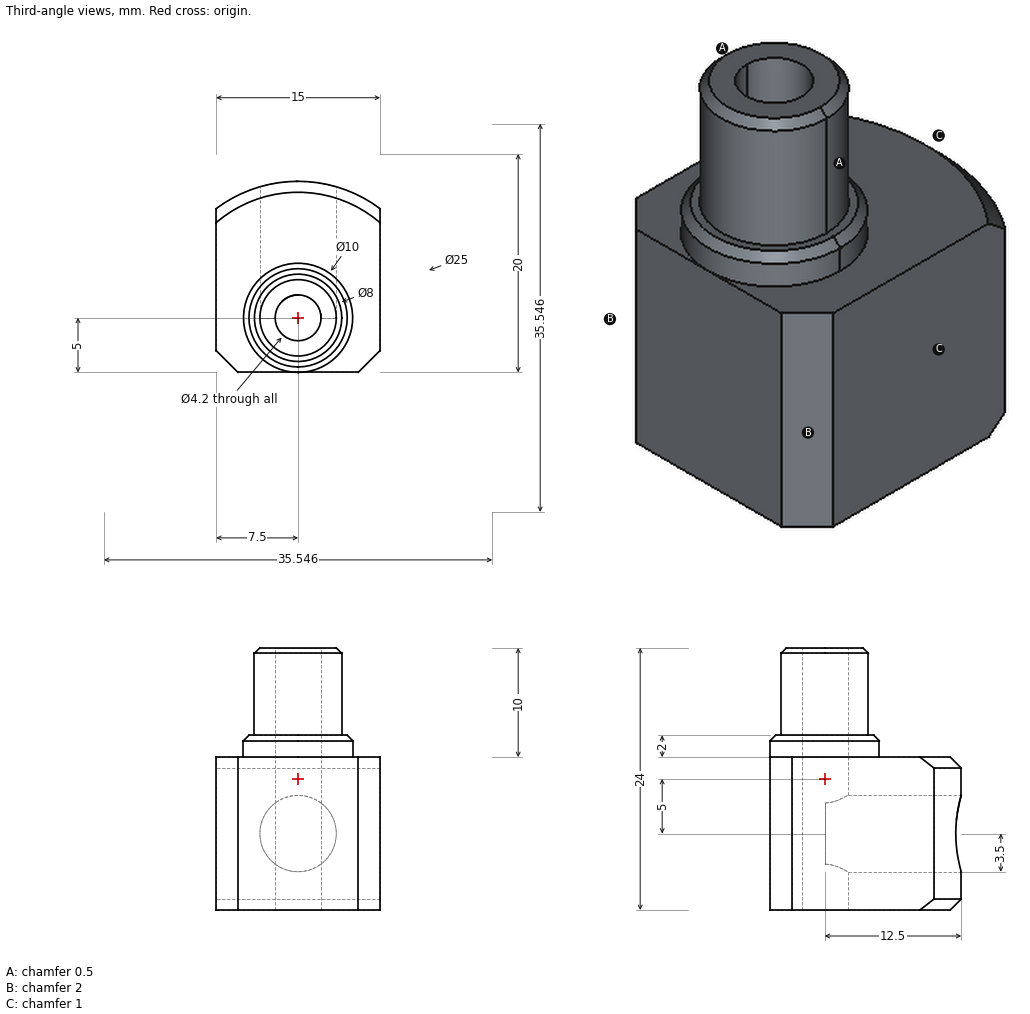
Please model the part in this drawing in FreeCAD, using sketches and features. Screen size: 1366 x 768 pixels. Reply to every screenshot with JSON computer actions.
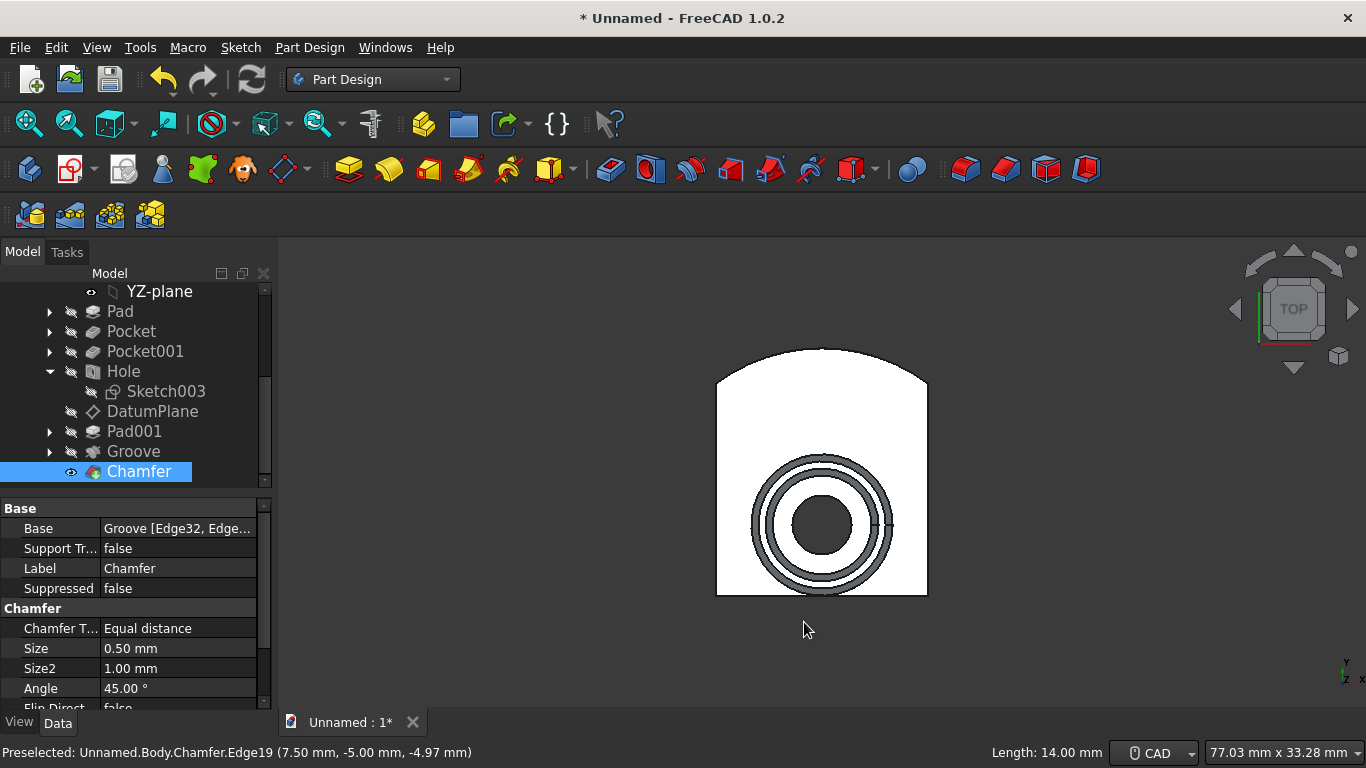
{"action": "key", "text": "0"}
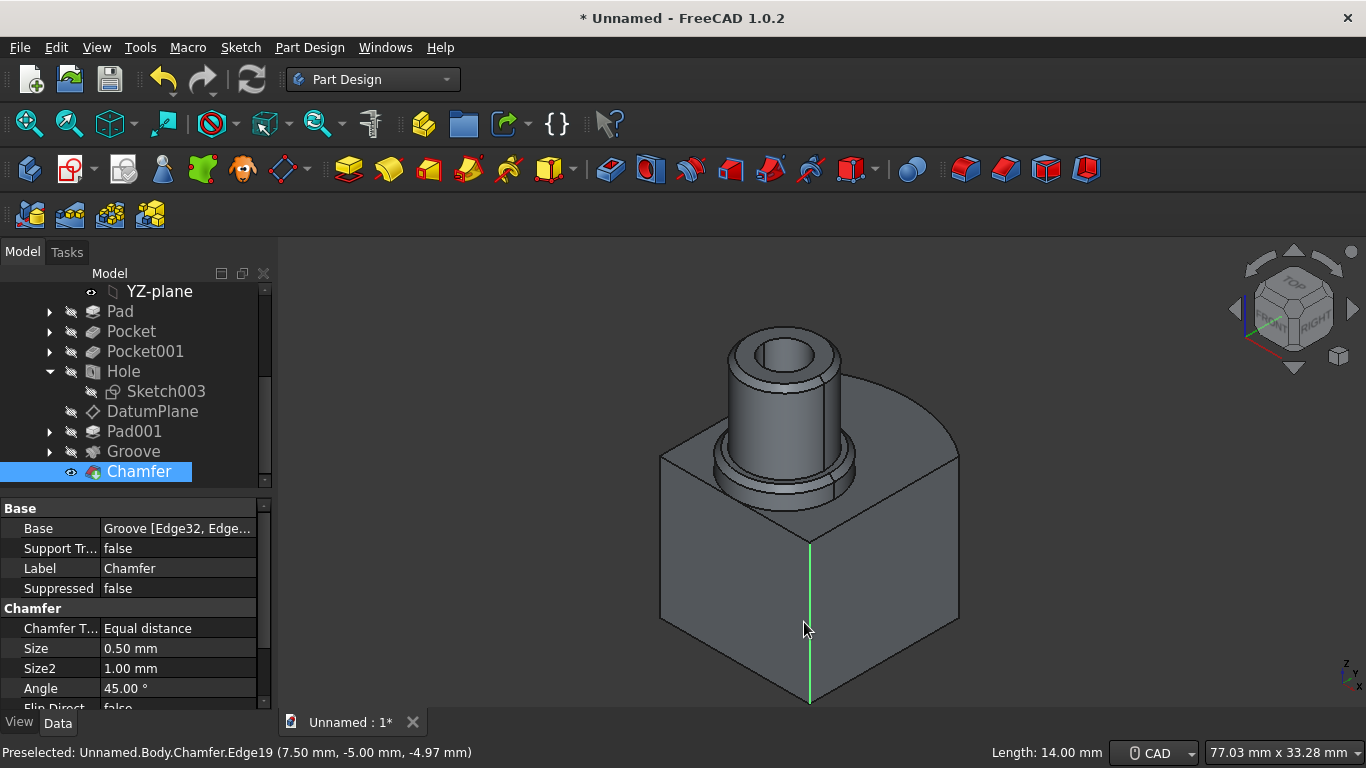
{"action": "key", "text": "1"}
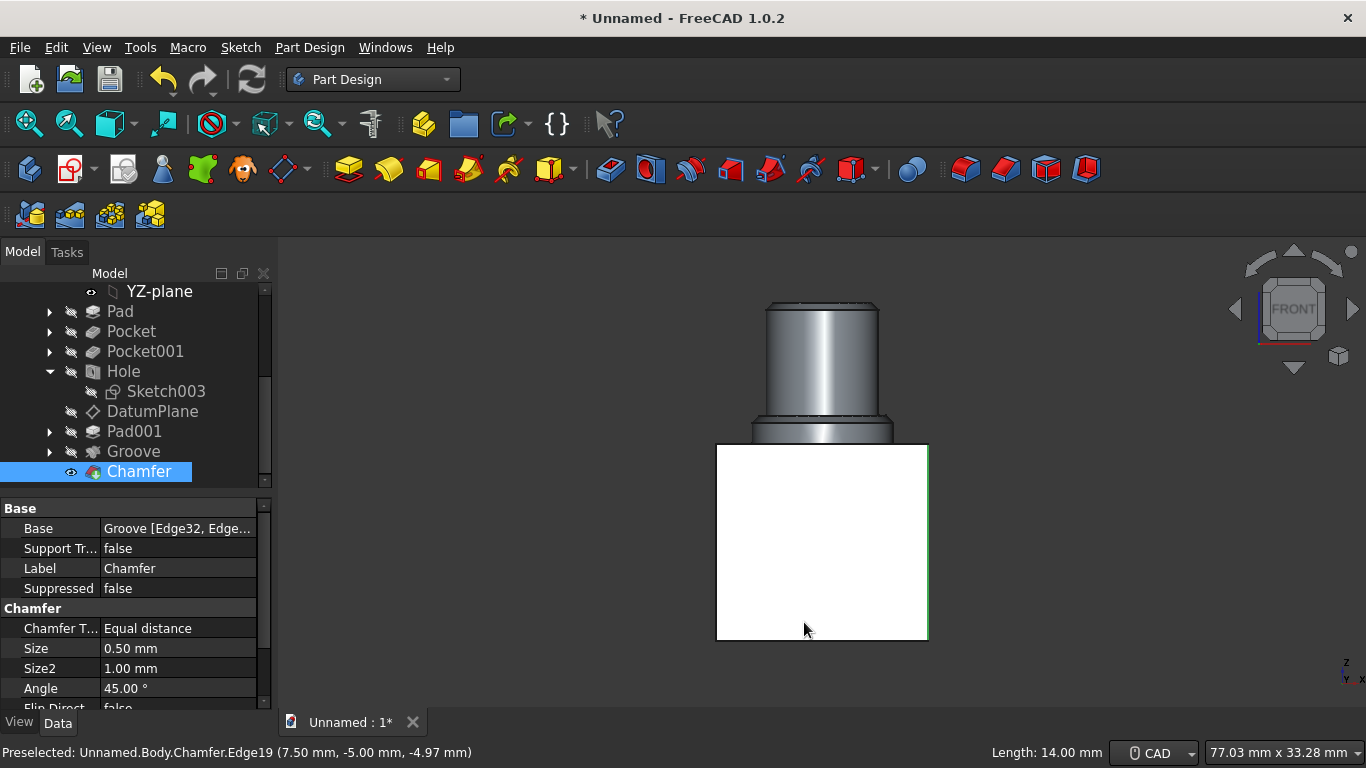
{"action": "left_click", "coordinate": [716, 542], "text": "ctrl"}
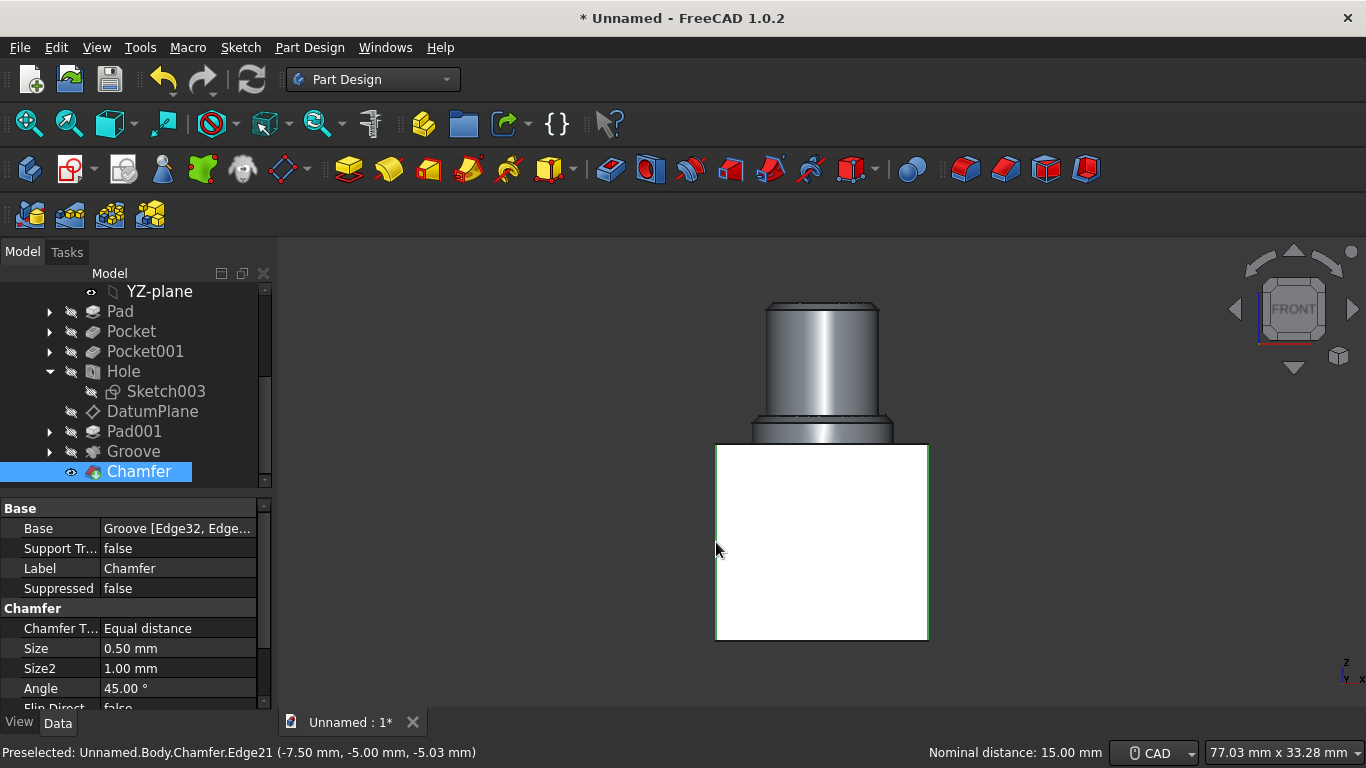
{"action": "left_click", "coordinate": [1006, 170]}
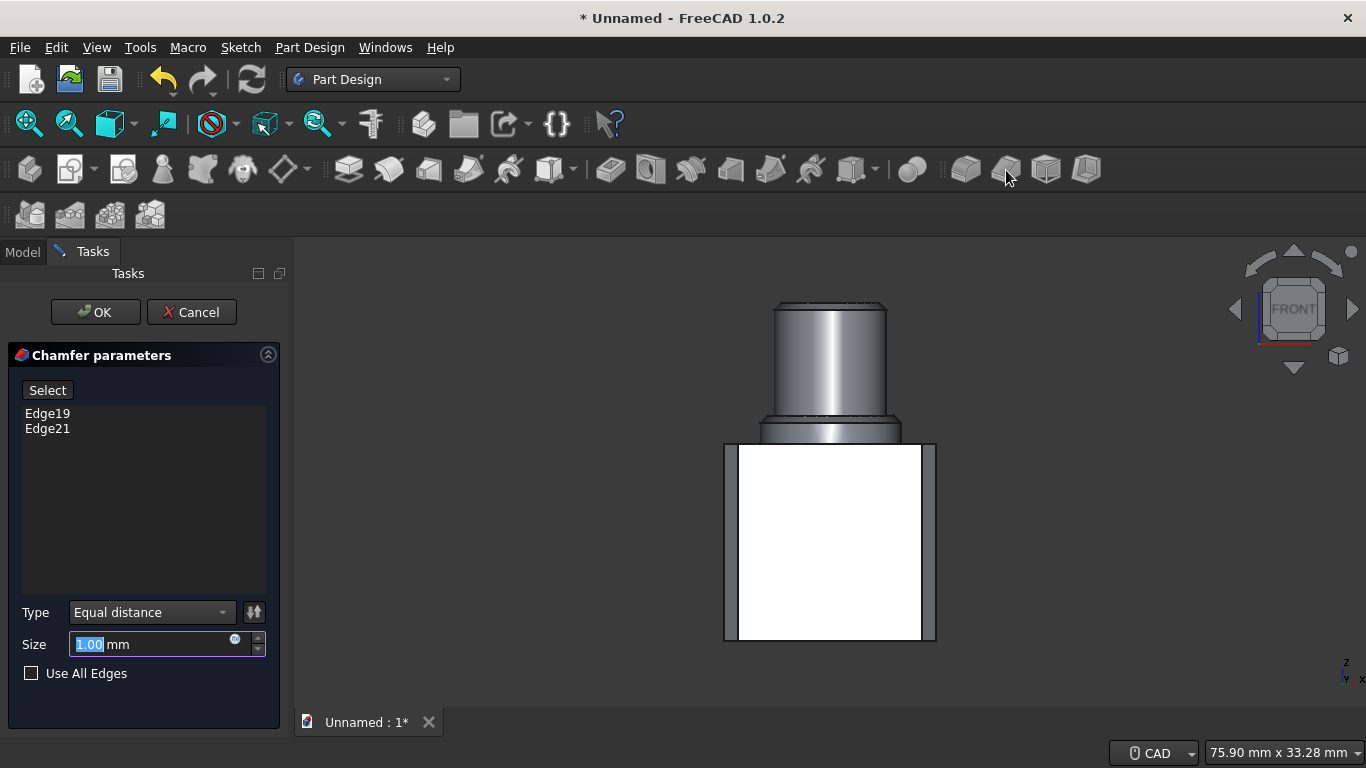
{"action": "type", "text": "2"}
{"action": "key", "text": "Tab"}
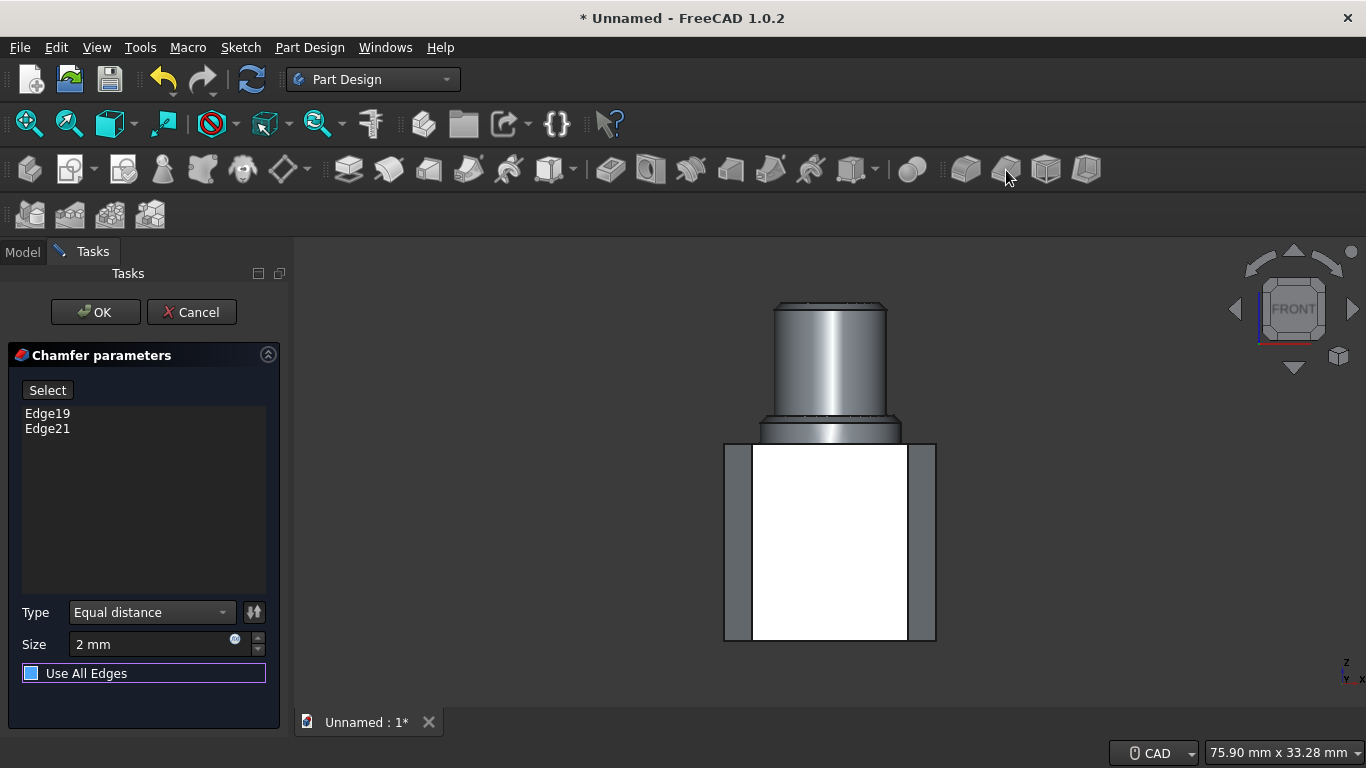
{"action": "left_click", "coordinate": [96, 312]}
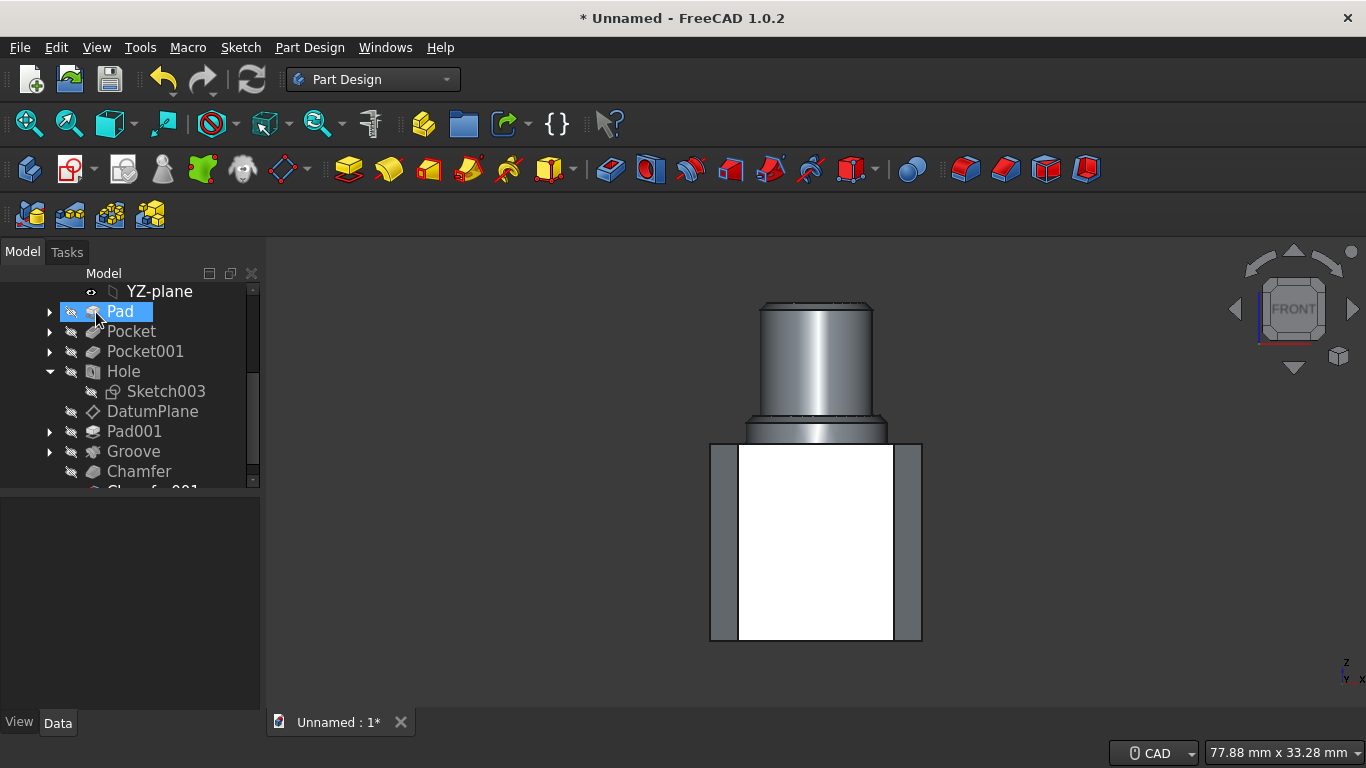
{"action": "key", "text": "0"}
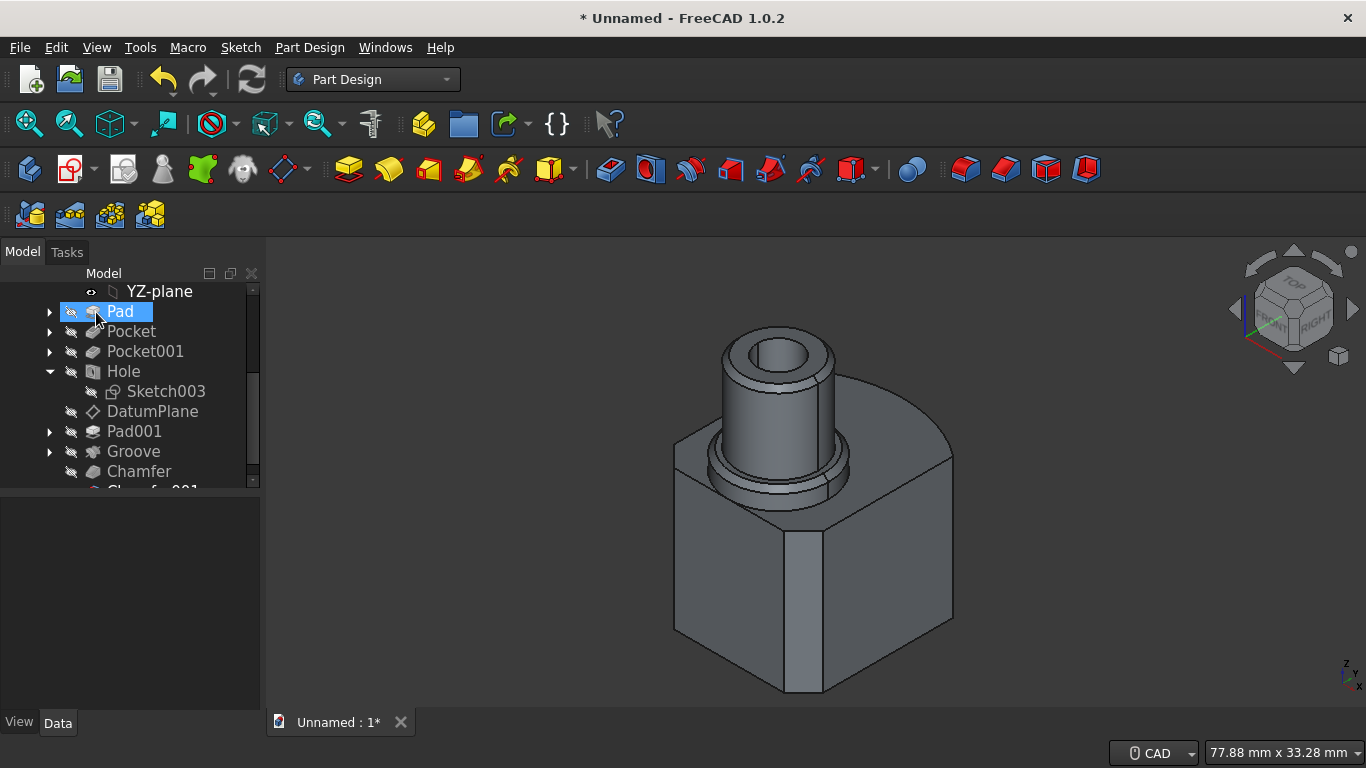
{"action": "key", "text": "2"}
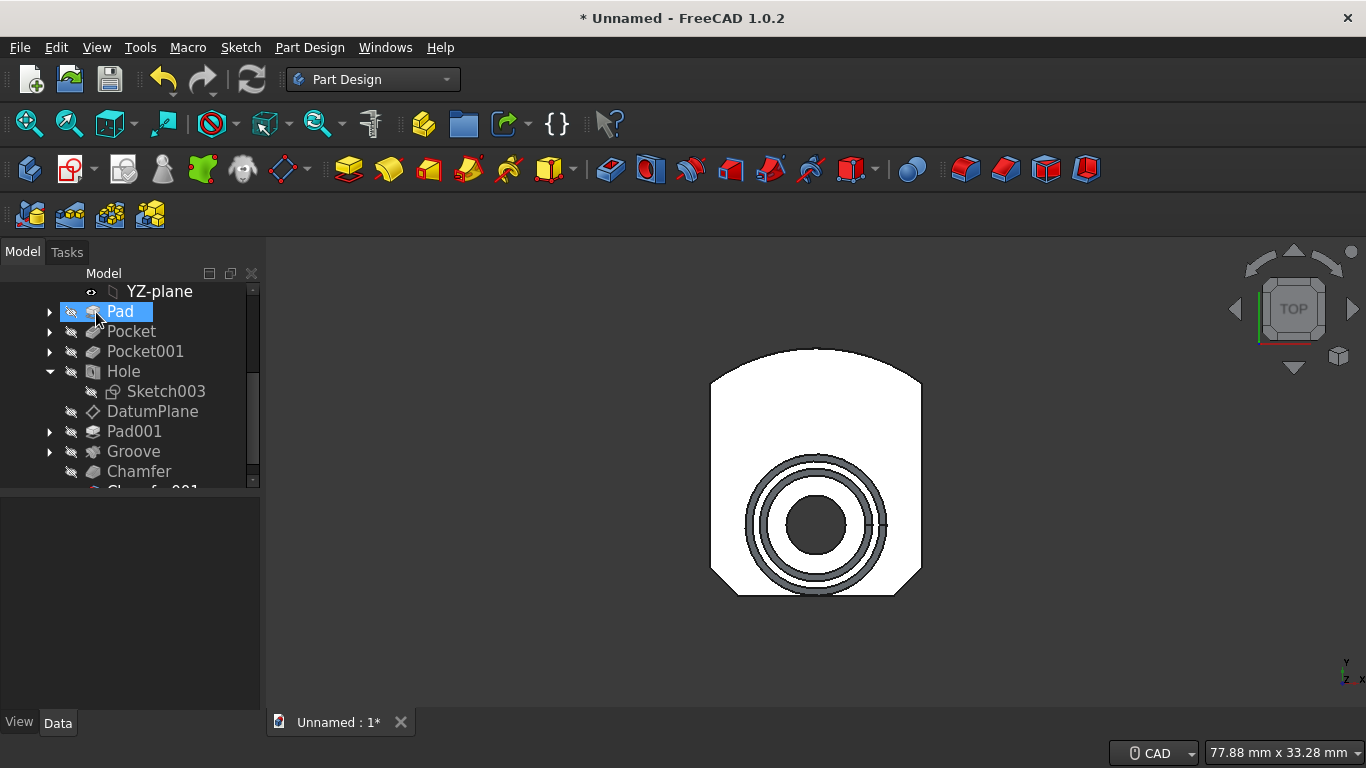
{"action": "left_click", "coordinate": [816, 347]}